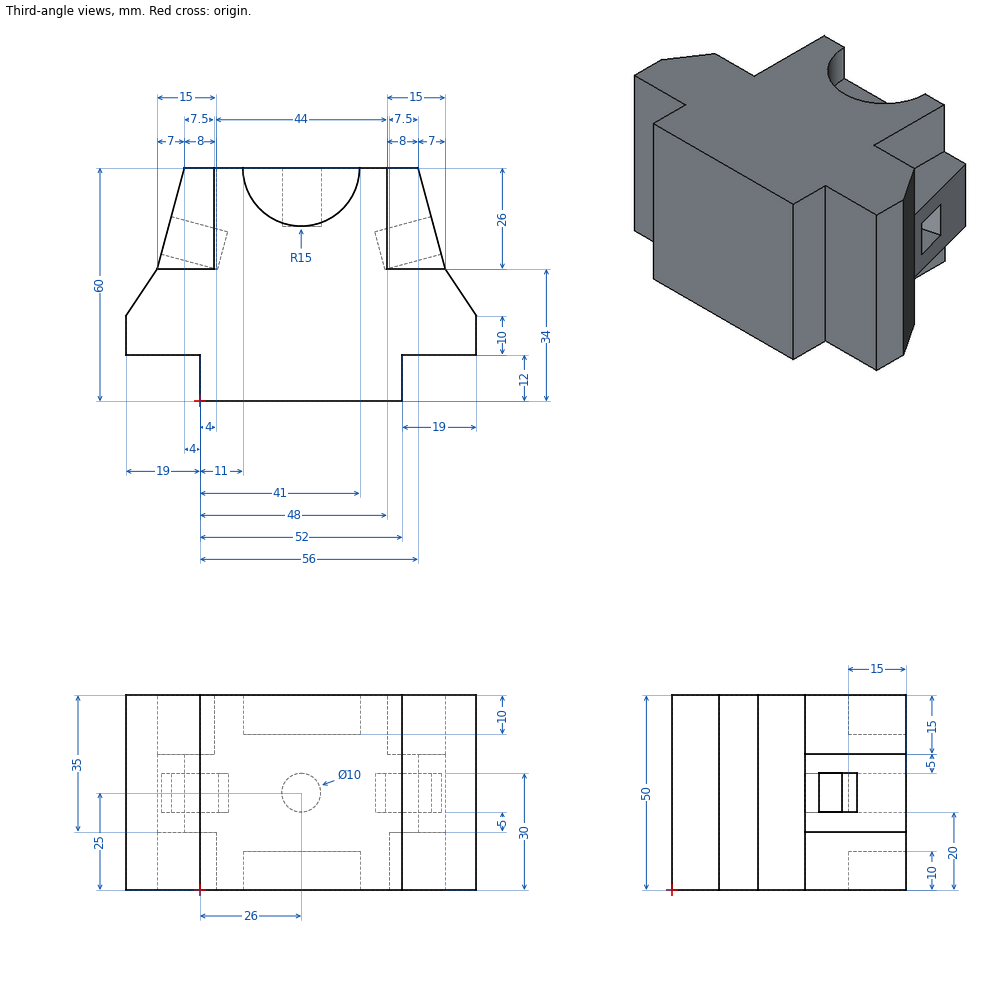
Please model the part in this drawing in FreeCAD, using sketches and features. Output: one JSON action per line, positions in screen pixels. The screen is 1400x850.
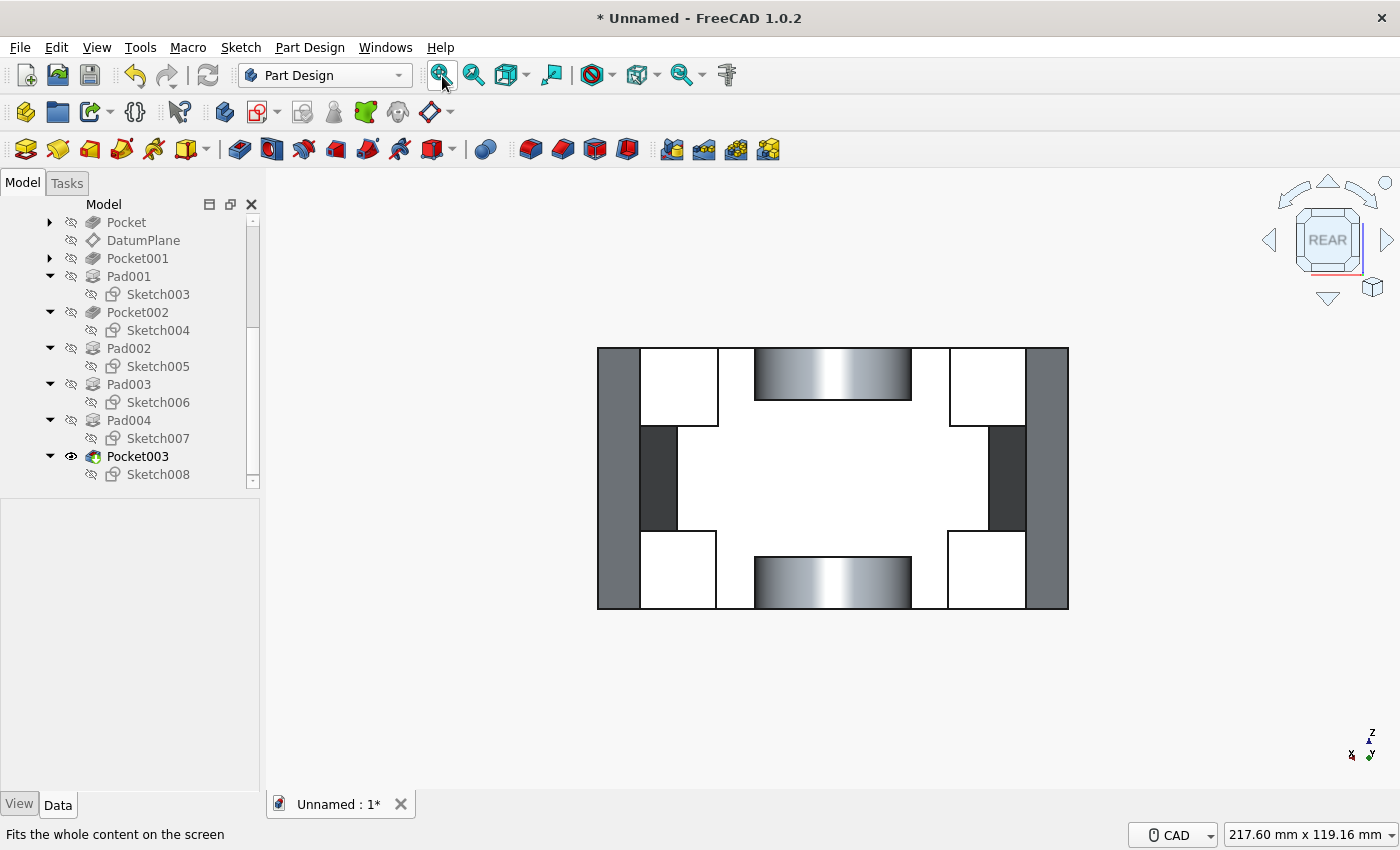
{"action": "left_click", "coordinate": [788, 478]}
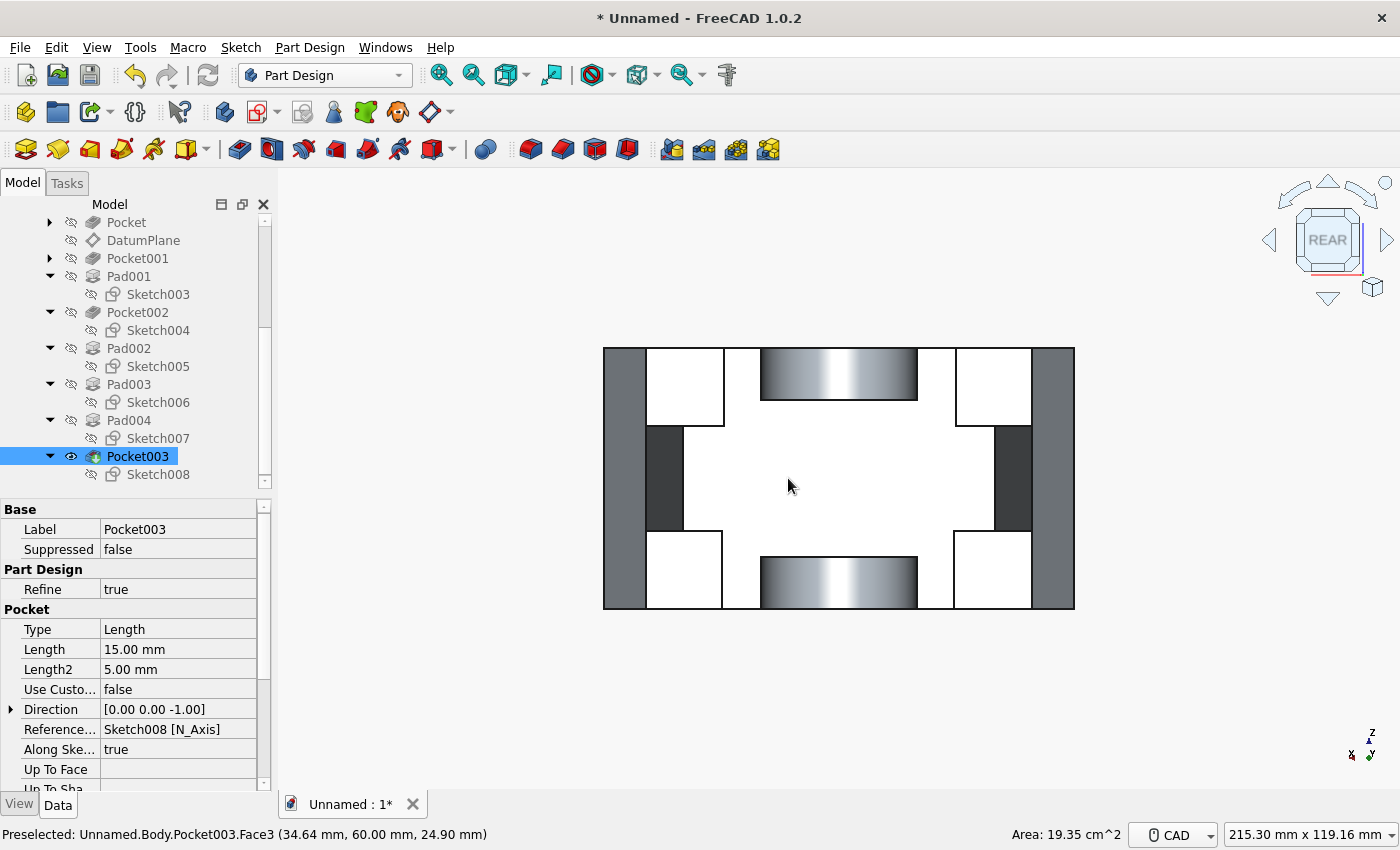
{"action": "left_click", "coordinate": [258, 112]}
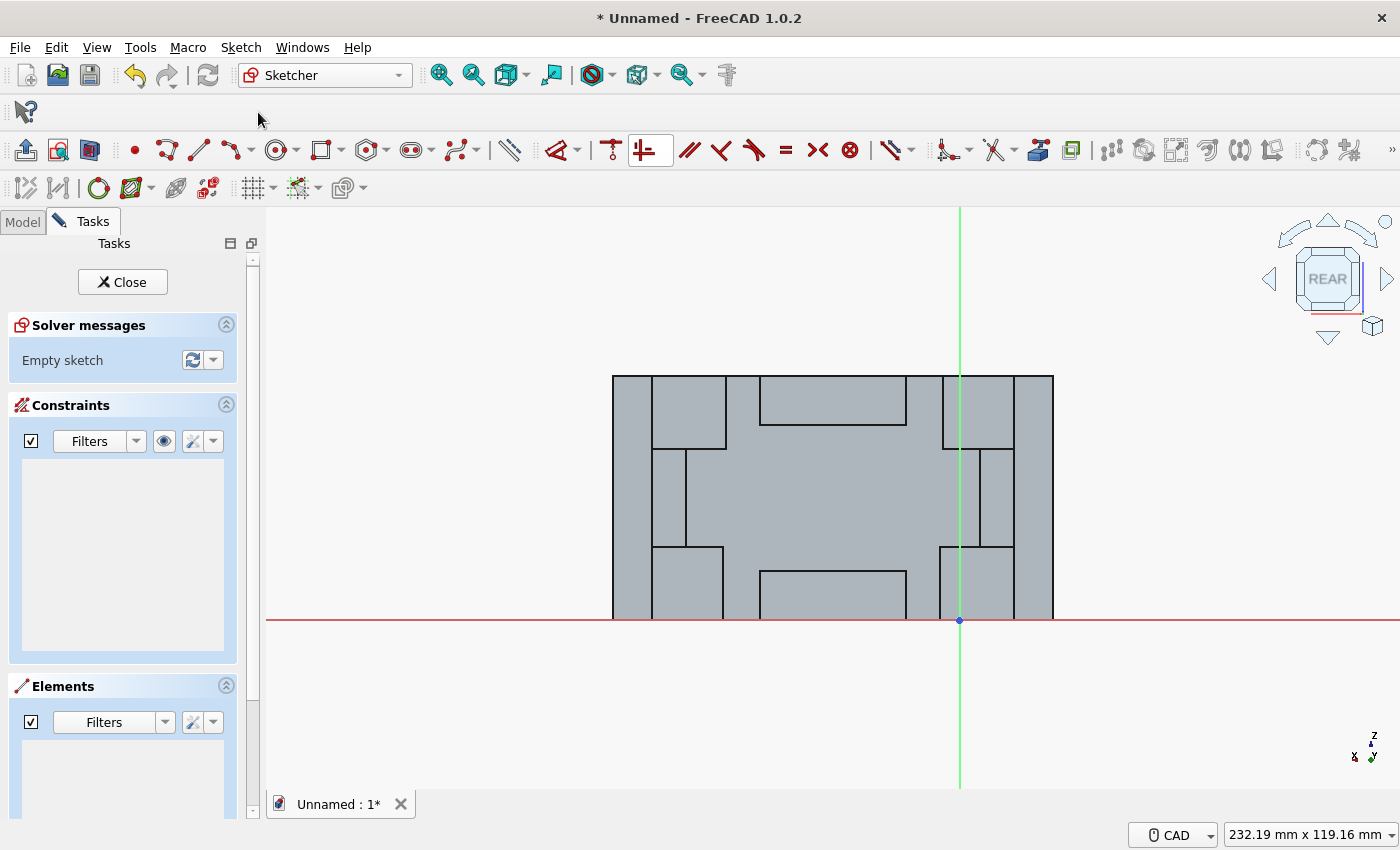
{"action": "scroll", "coordinate": [844, 498], "scroll_direction": "up", "scroll_amount": 10}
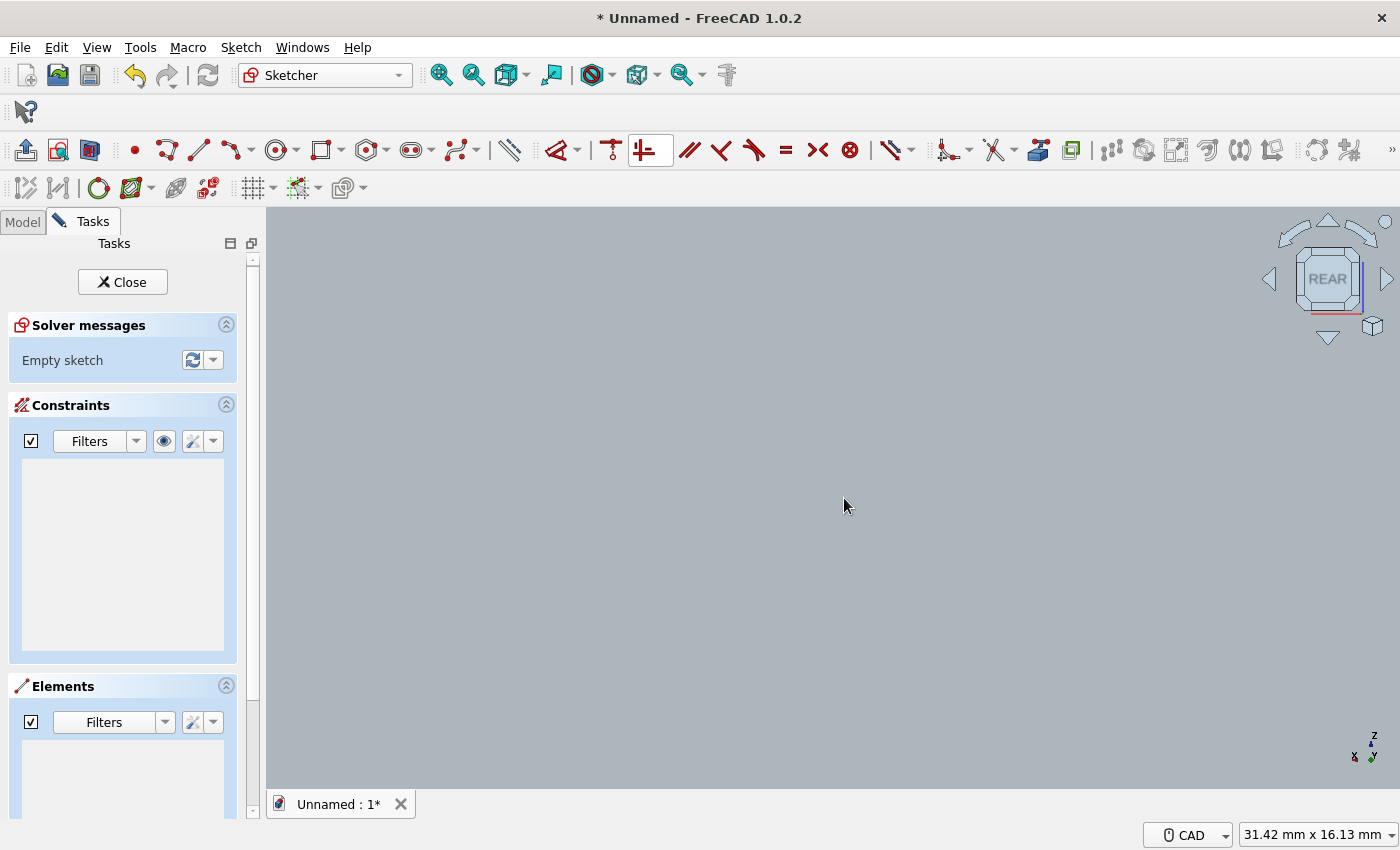
{"action": "left_click", "coordinate": [276, 150]}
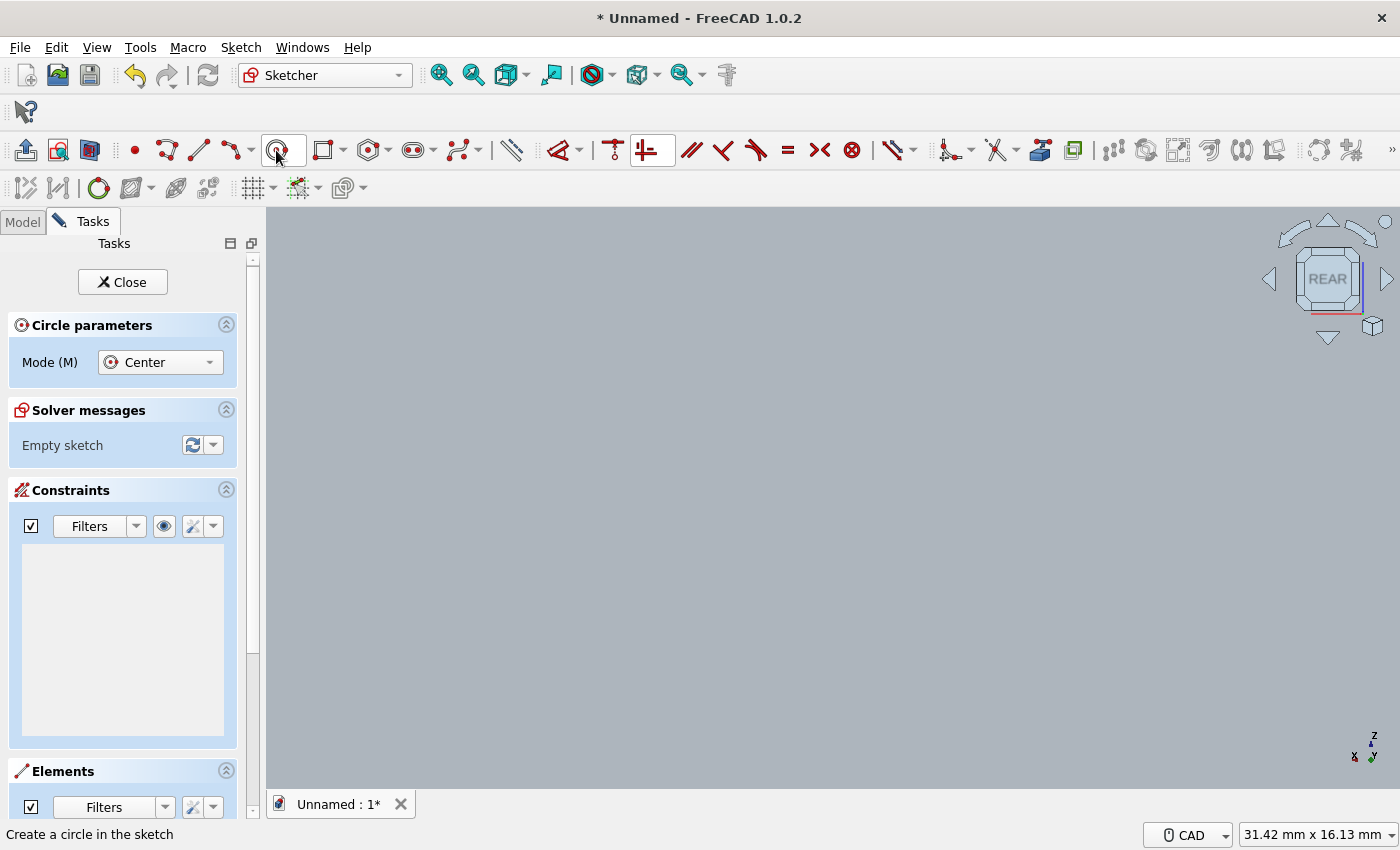
{"action": "left_click", "coordinate": [759, 495]}
{"action": "left_click", "coordinate": [887, 367]}
{"action": "key", "text": "Escape"}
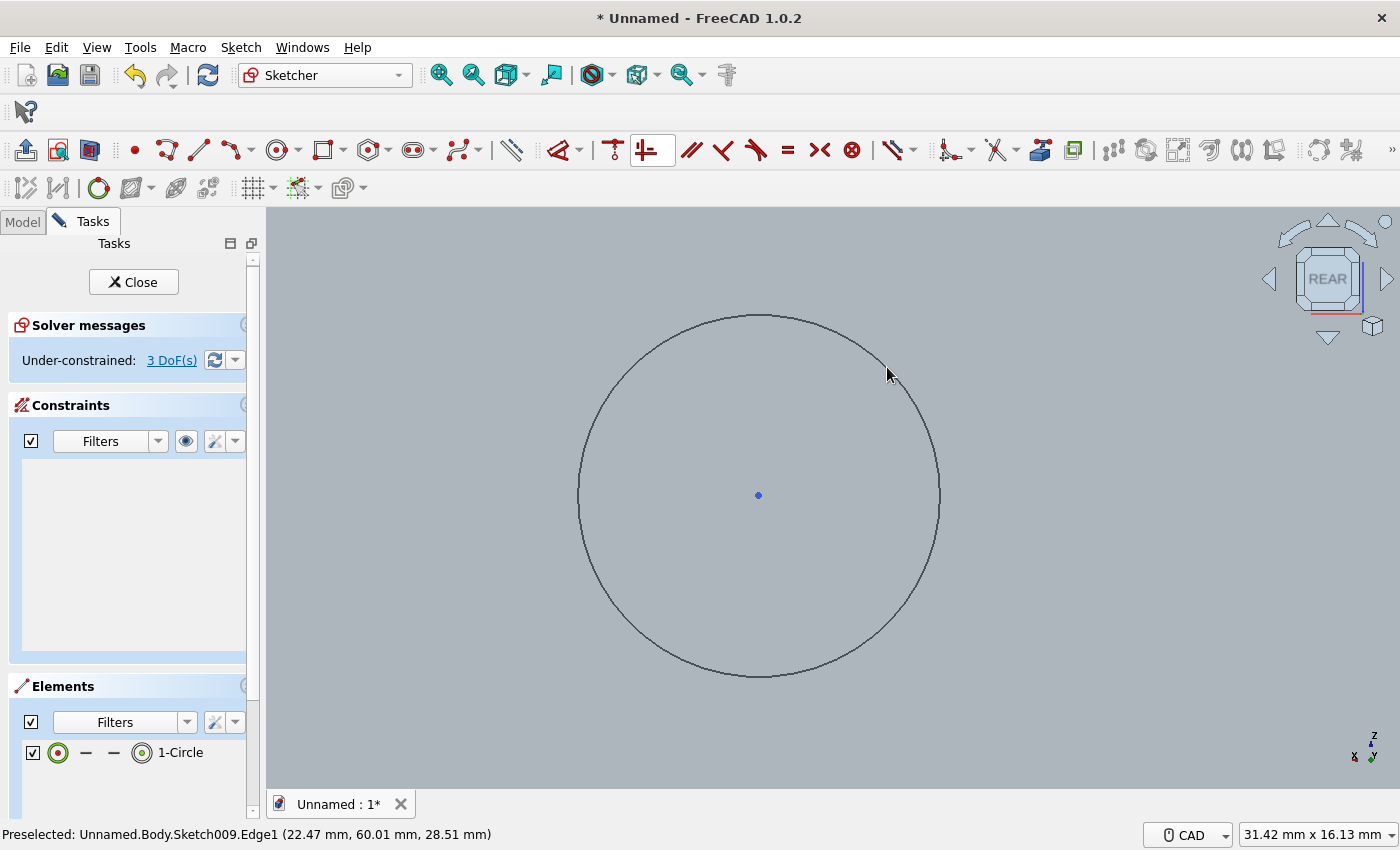
{"action": "left_click", "coordinate": [558, 150]}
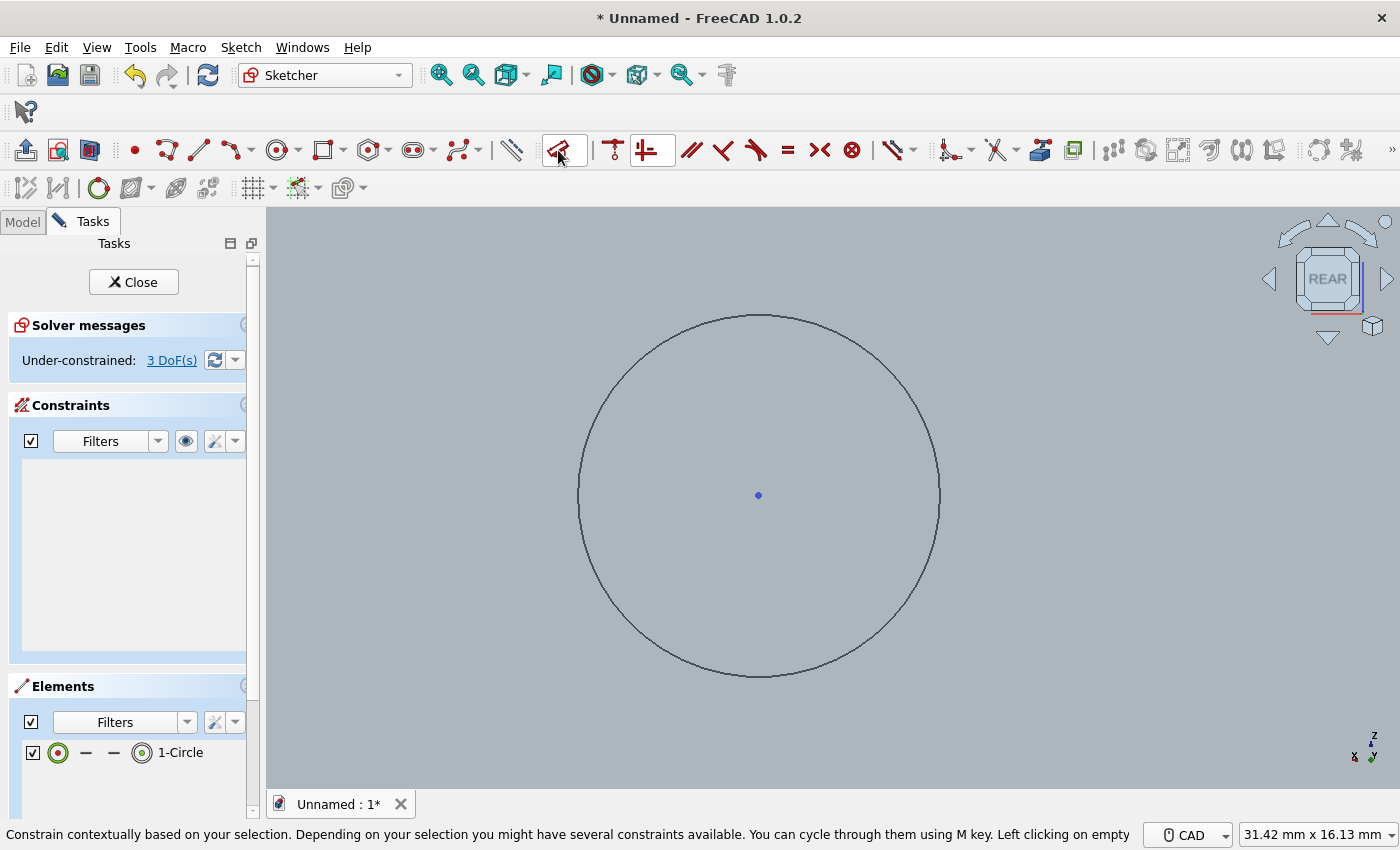
{"action": "left_click", "coordinate": [887, 368]}
{"action": "left_click", "coordinate": [910, 345]}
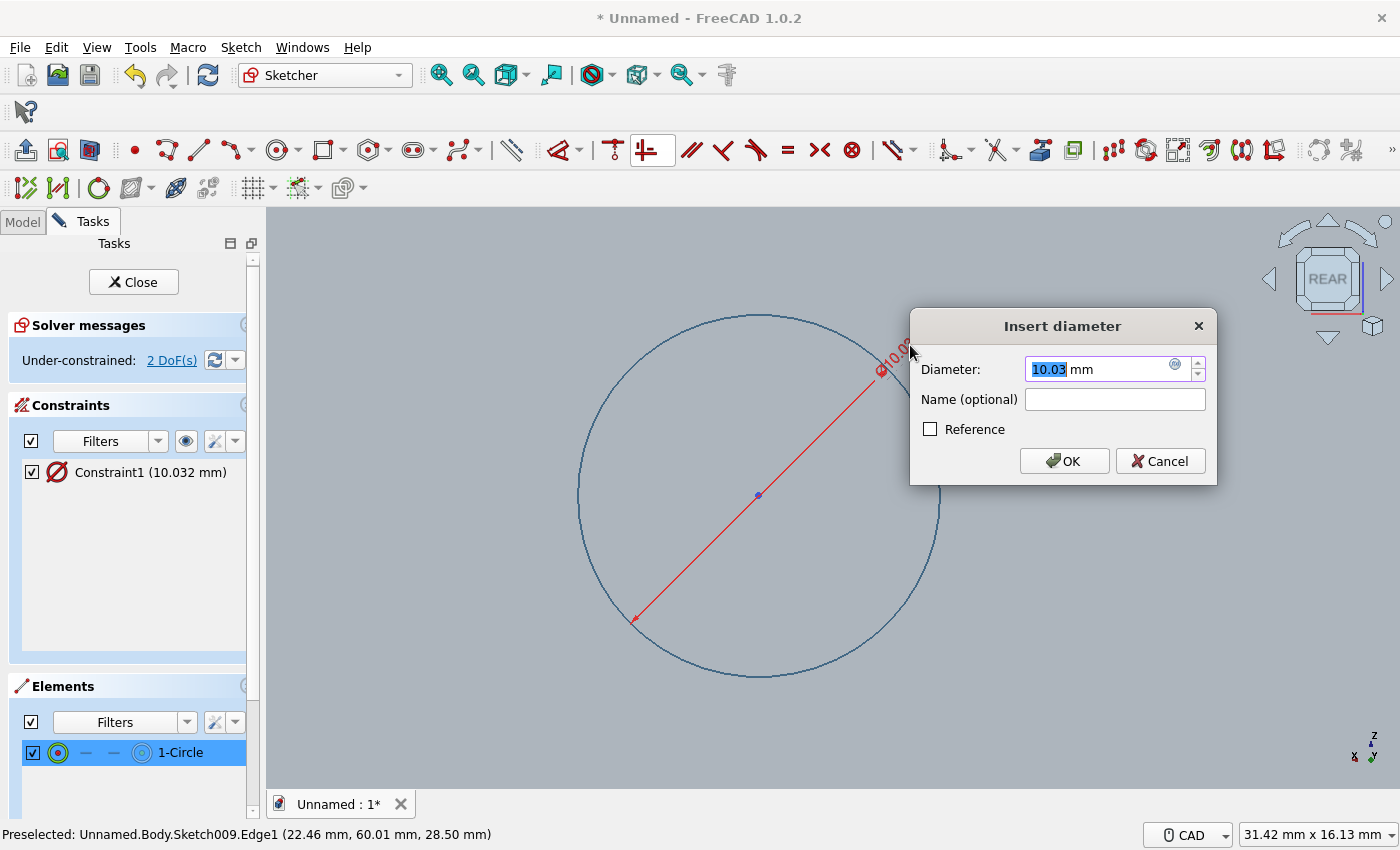
{"action": "type", "text": "10"}
{"action": "key", "text": "Return"}